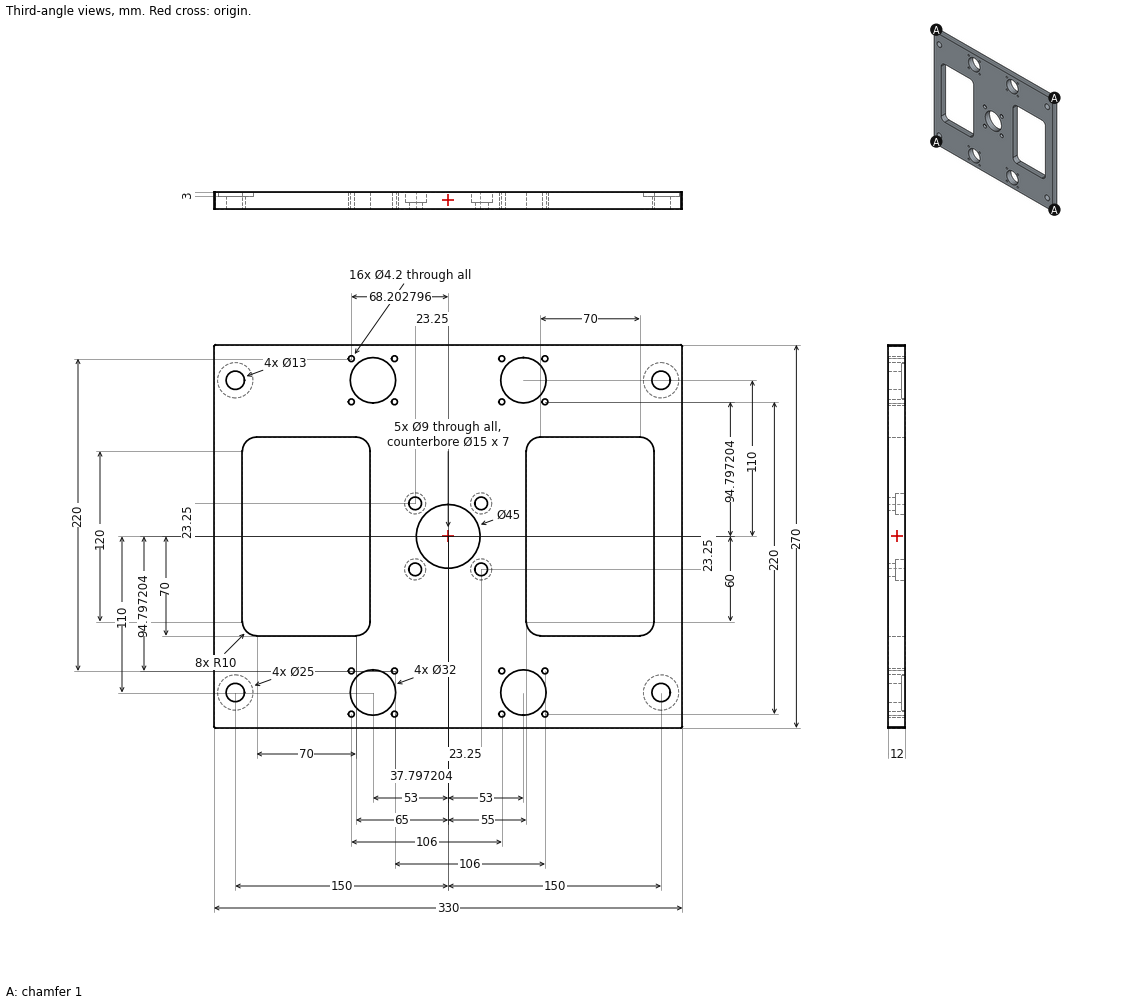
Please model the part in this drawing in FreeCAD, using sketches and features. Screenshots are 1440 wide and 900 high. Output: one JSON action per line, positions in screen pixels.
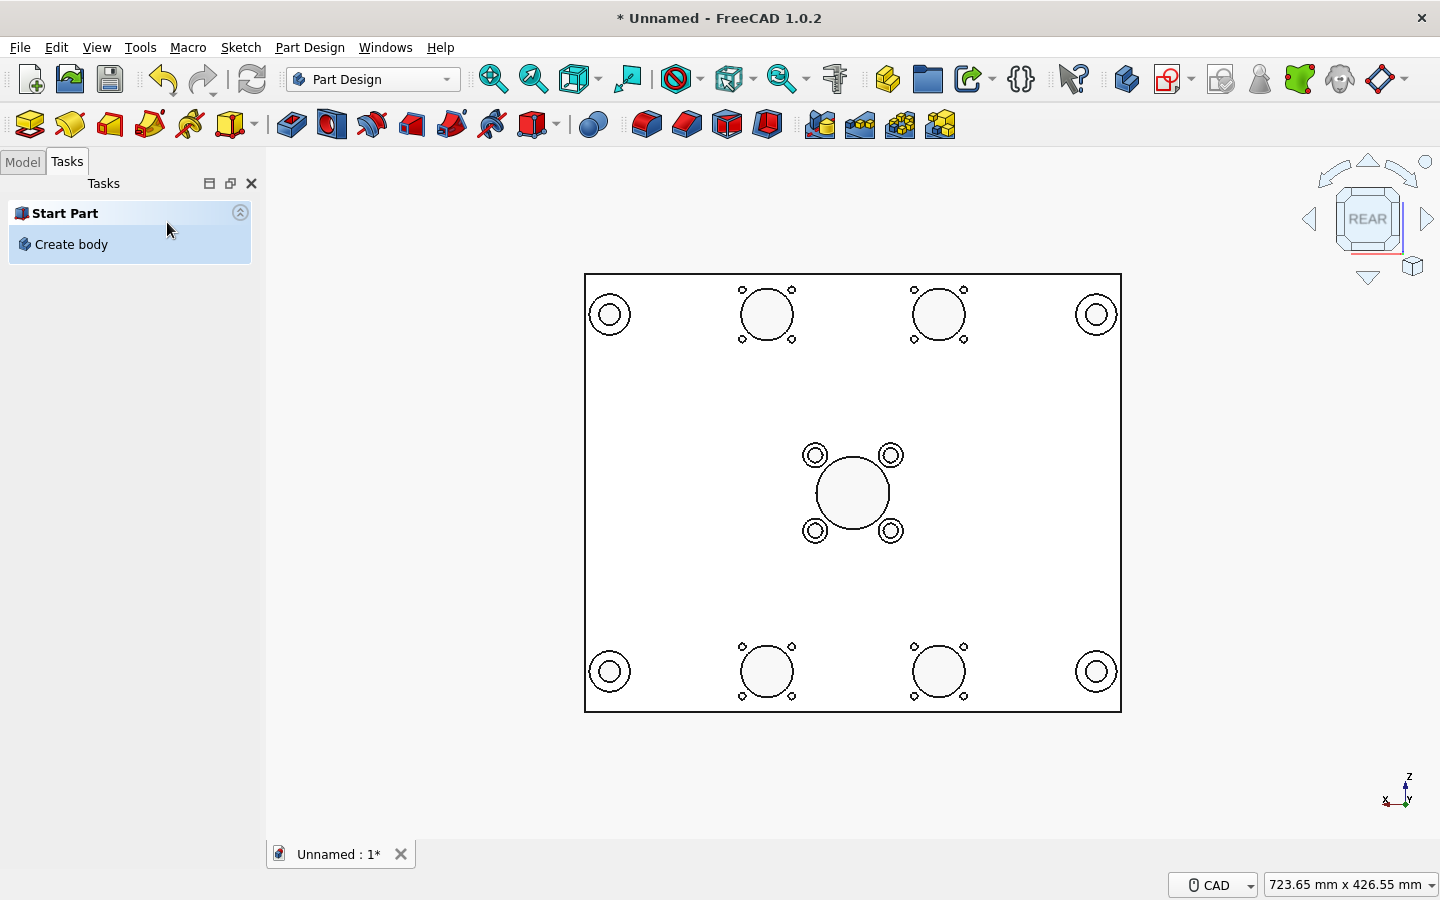
{"action": "scroll", "coordinate": [585, 273], "scroll_direction": "up", "scroll_amount": 4}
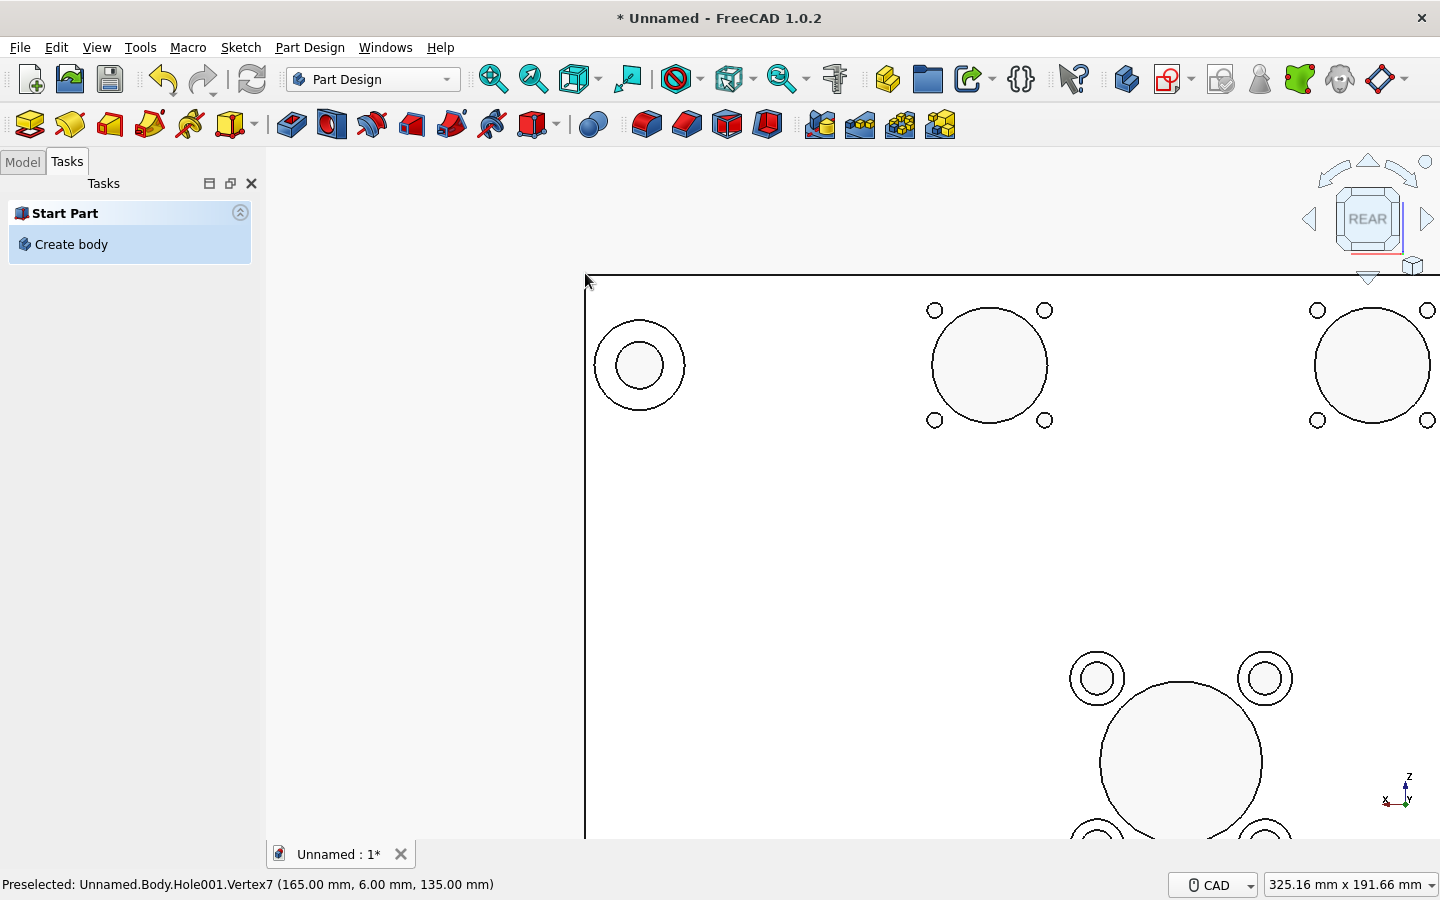
{"action": "left_click", "coordinate": [494, 80]}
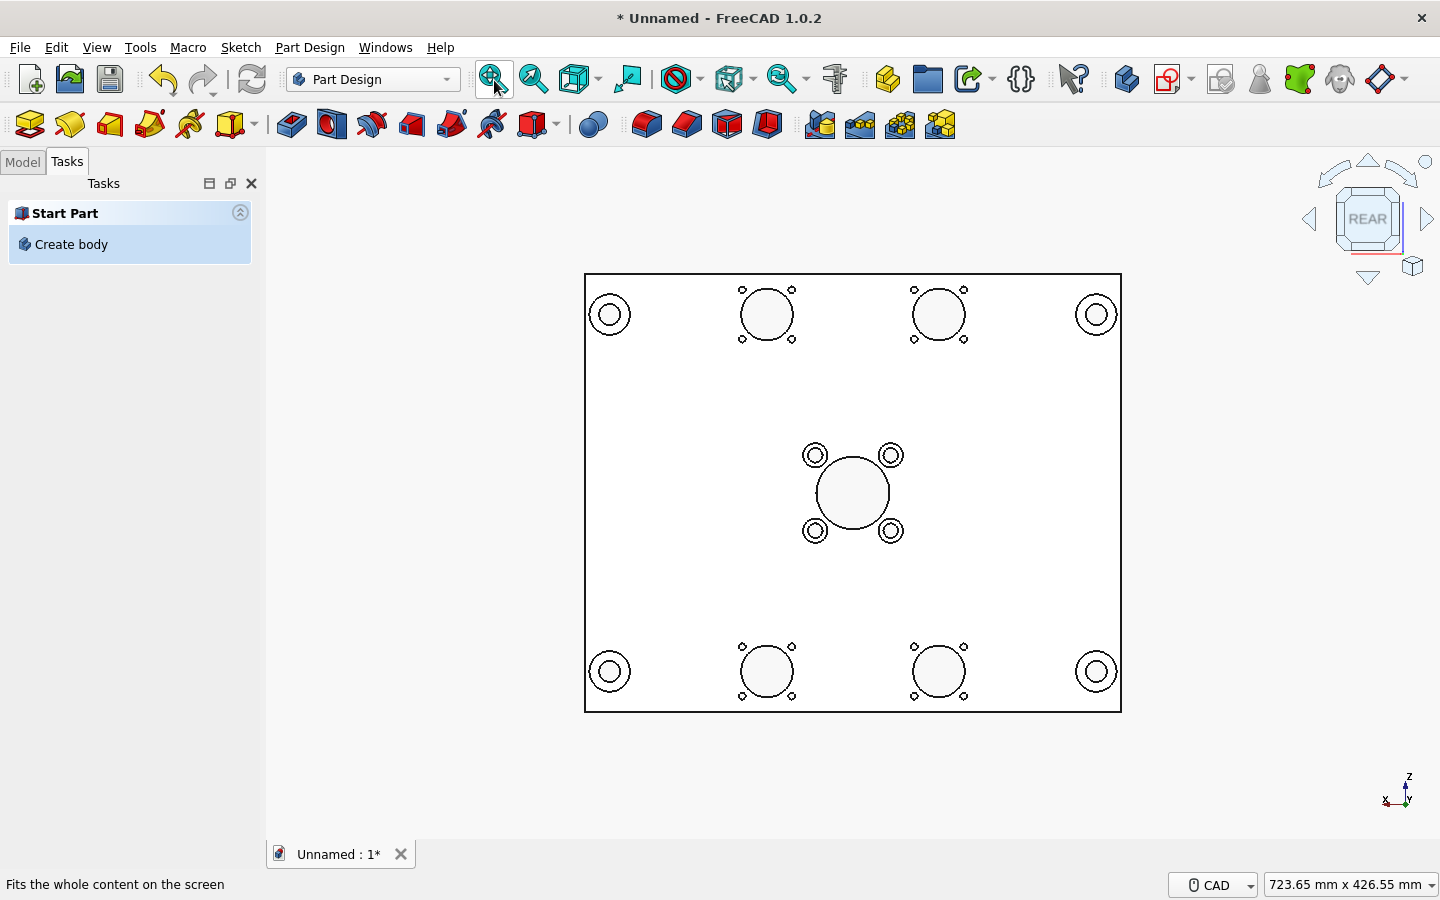
{"action": "key", "text": "0"}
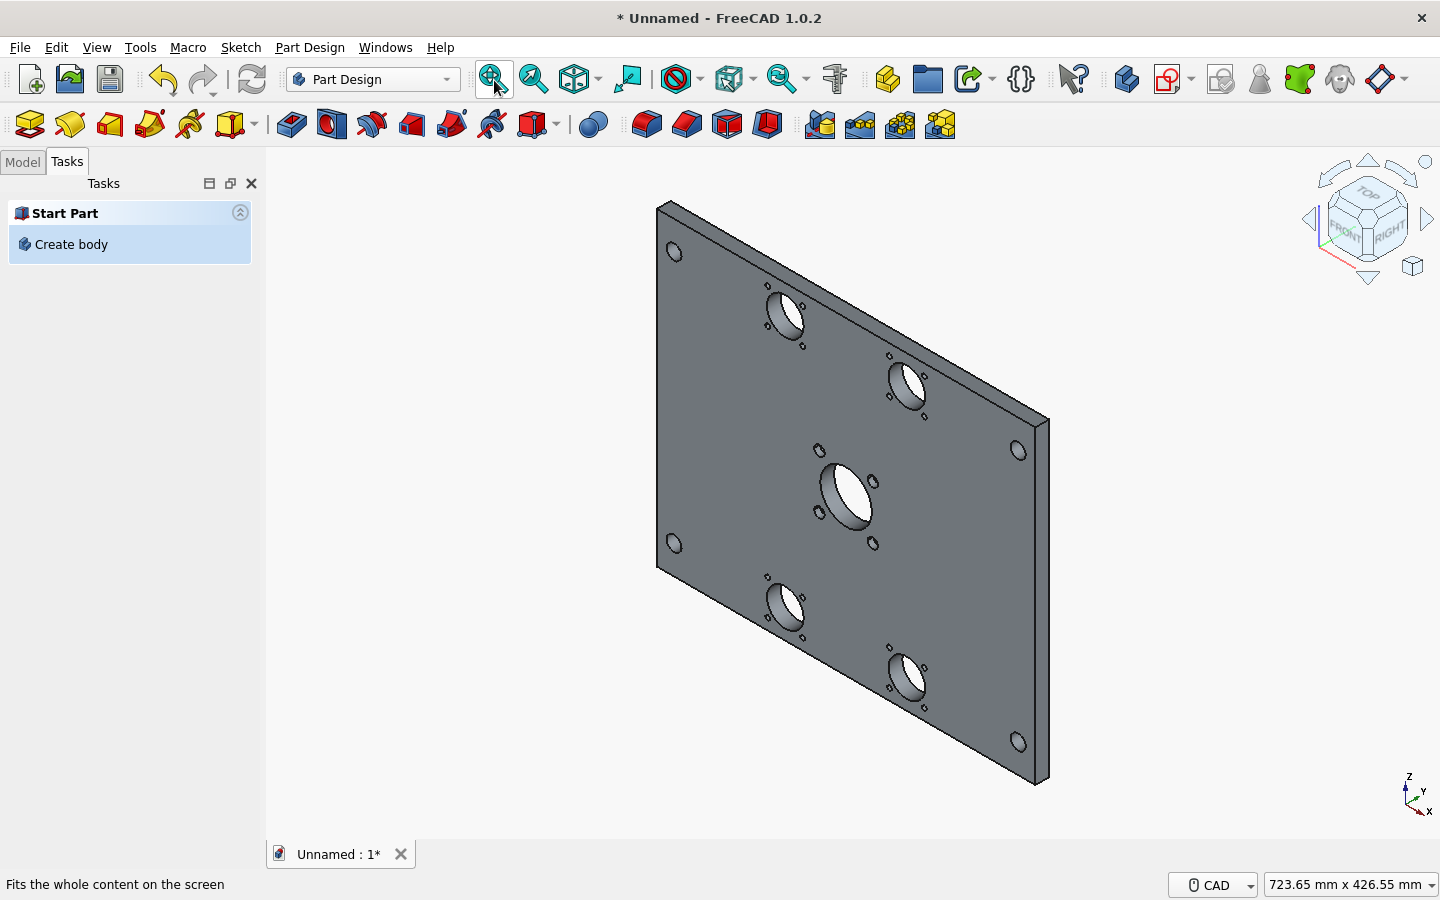
{"action": "left_click", "coordinate": [1042, 422]}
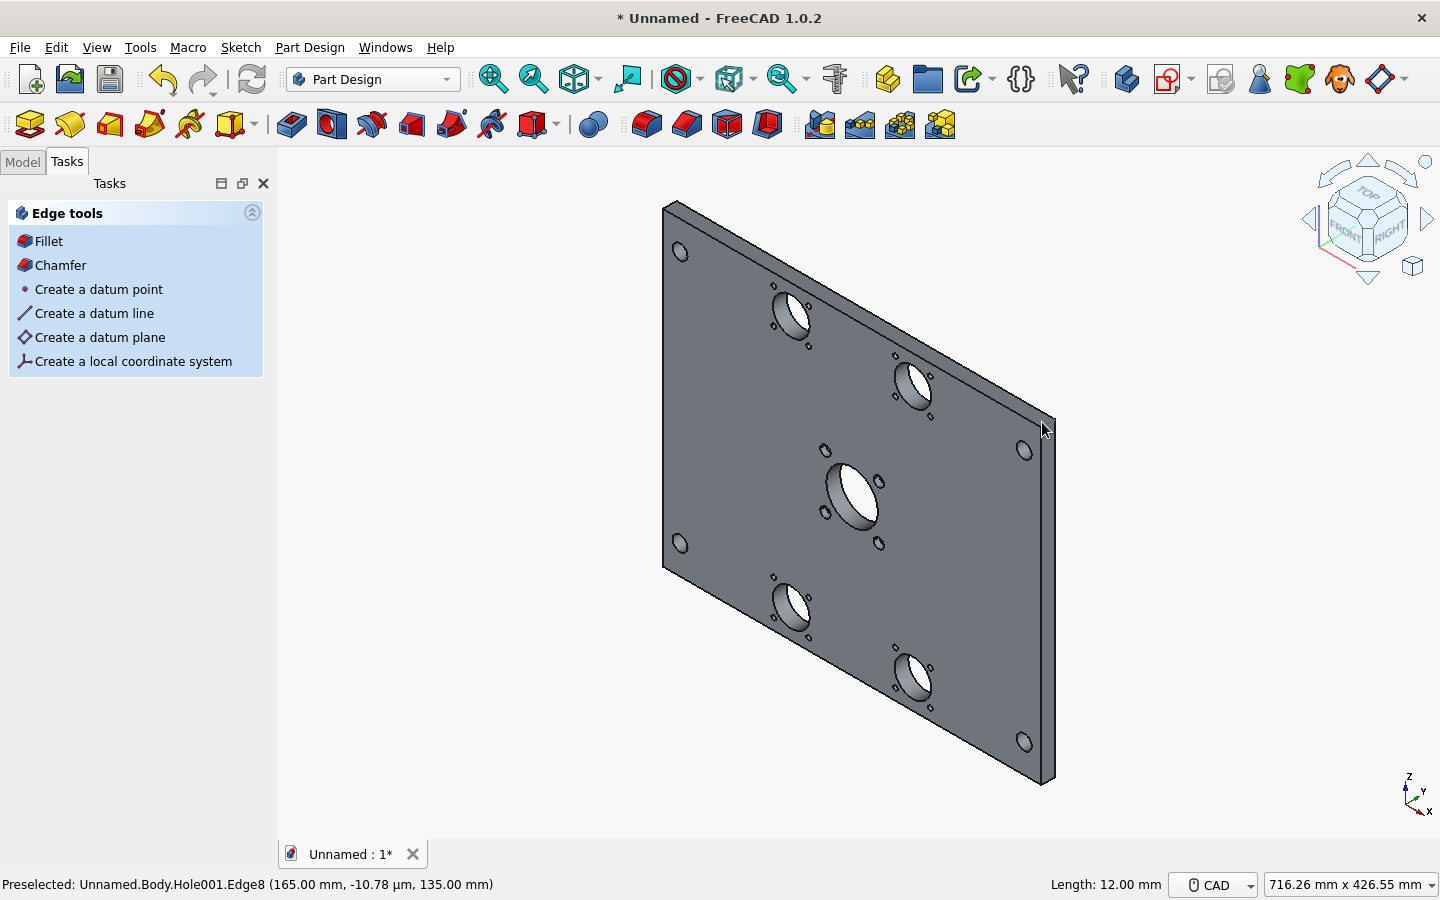
{"action": "scroll", "coordinate": [670, 204], "scroll_direction": "up", "scroll_amount": 4}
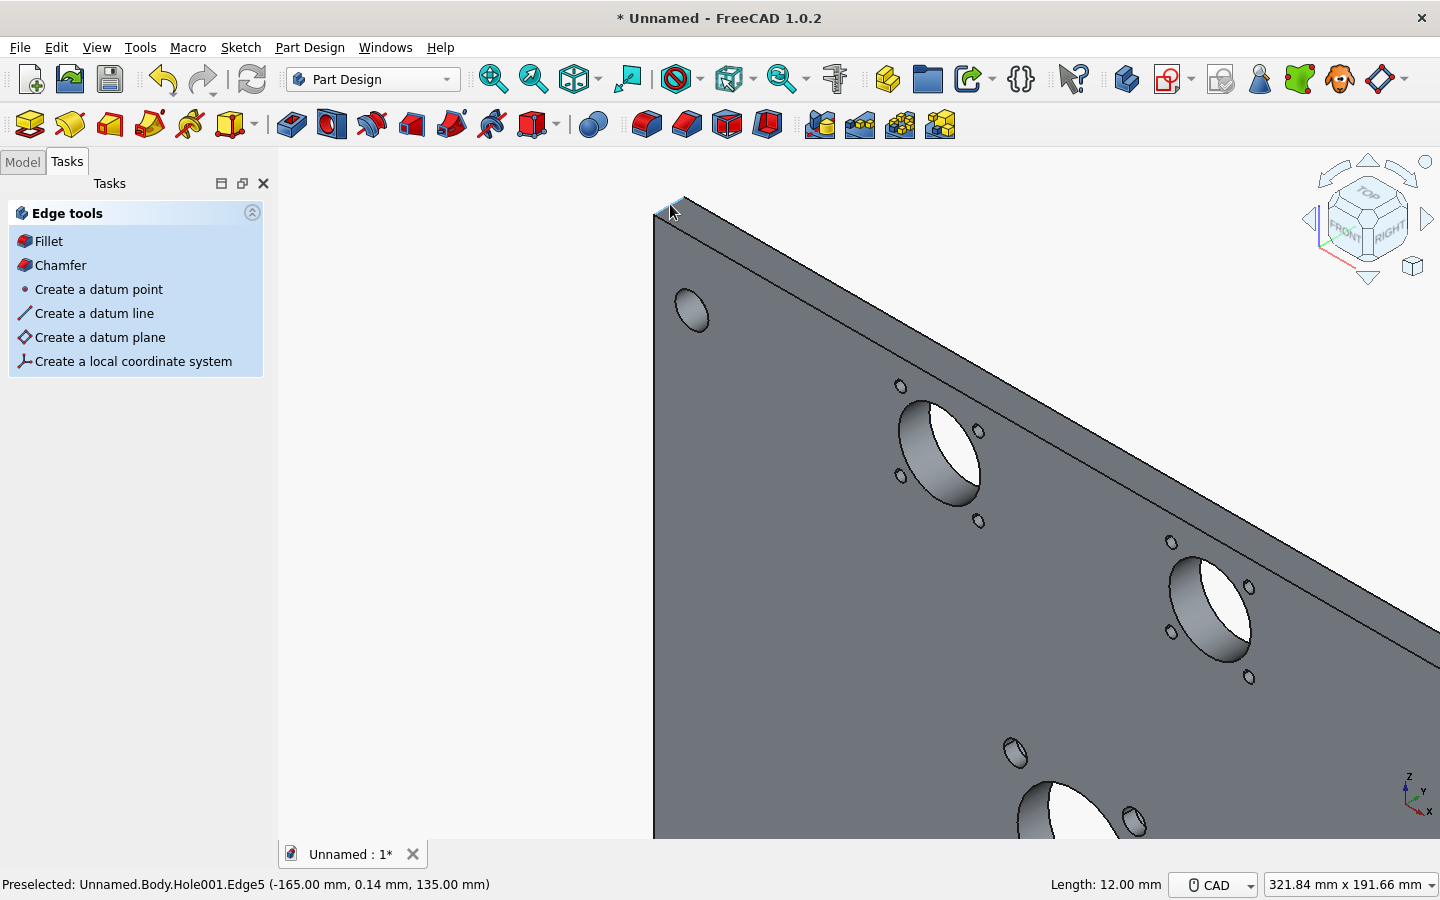
{"action": "left_click", "coordinate": [494, 80]}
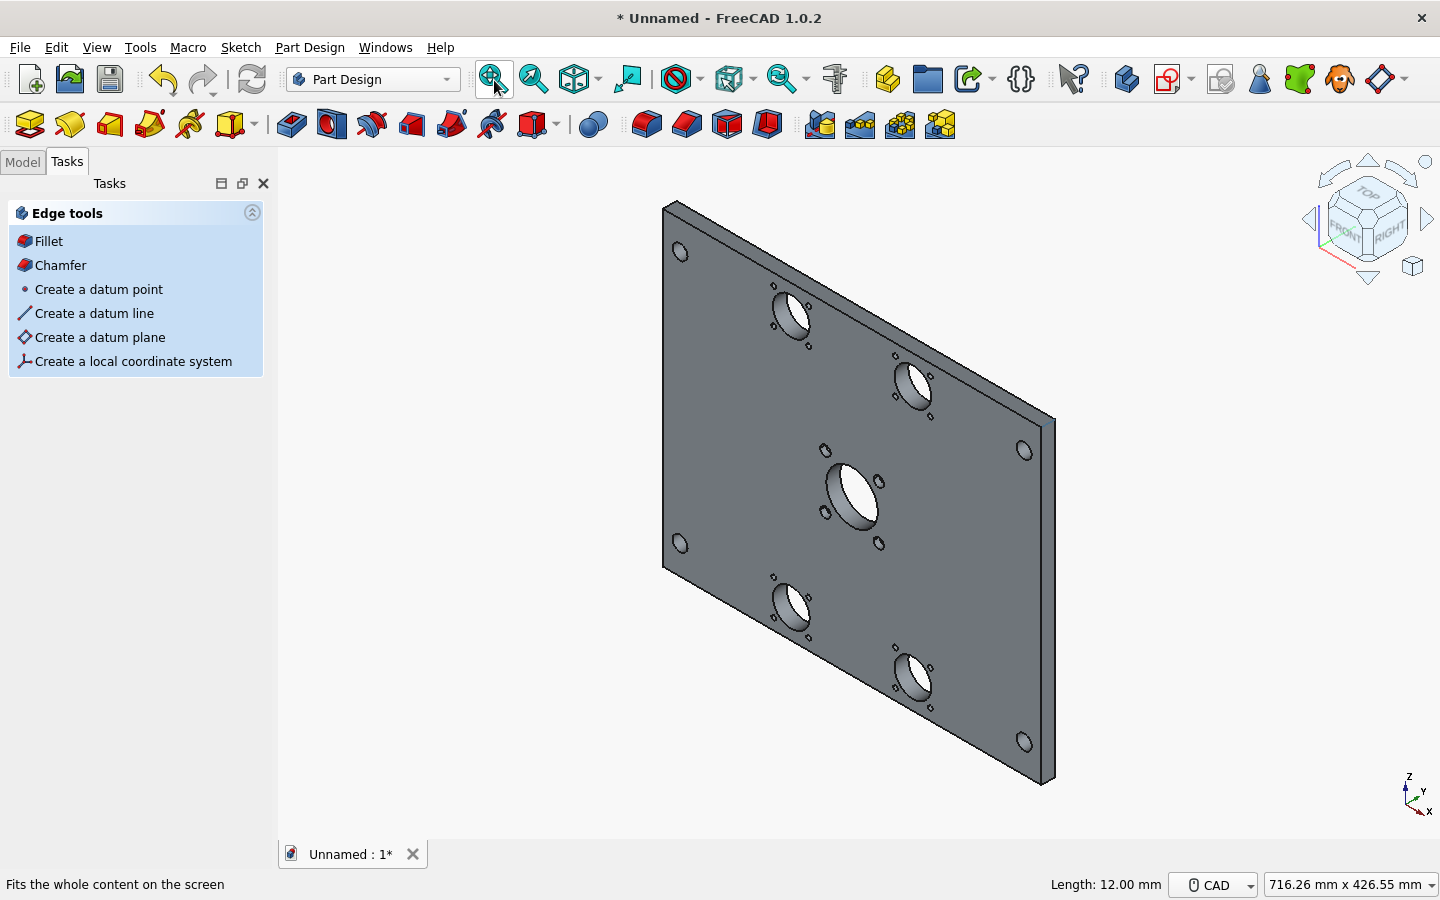
{"action": "key", "text": "2"}